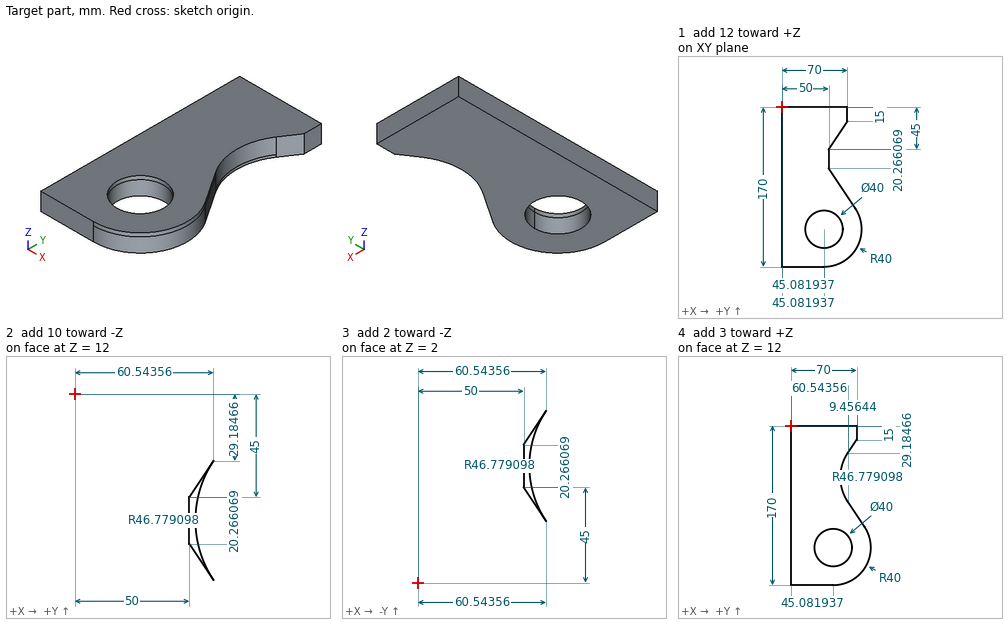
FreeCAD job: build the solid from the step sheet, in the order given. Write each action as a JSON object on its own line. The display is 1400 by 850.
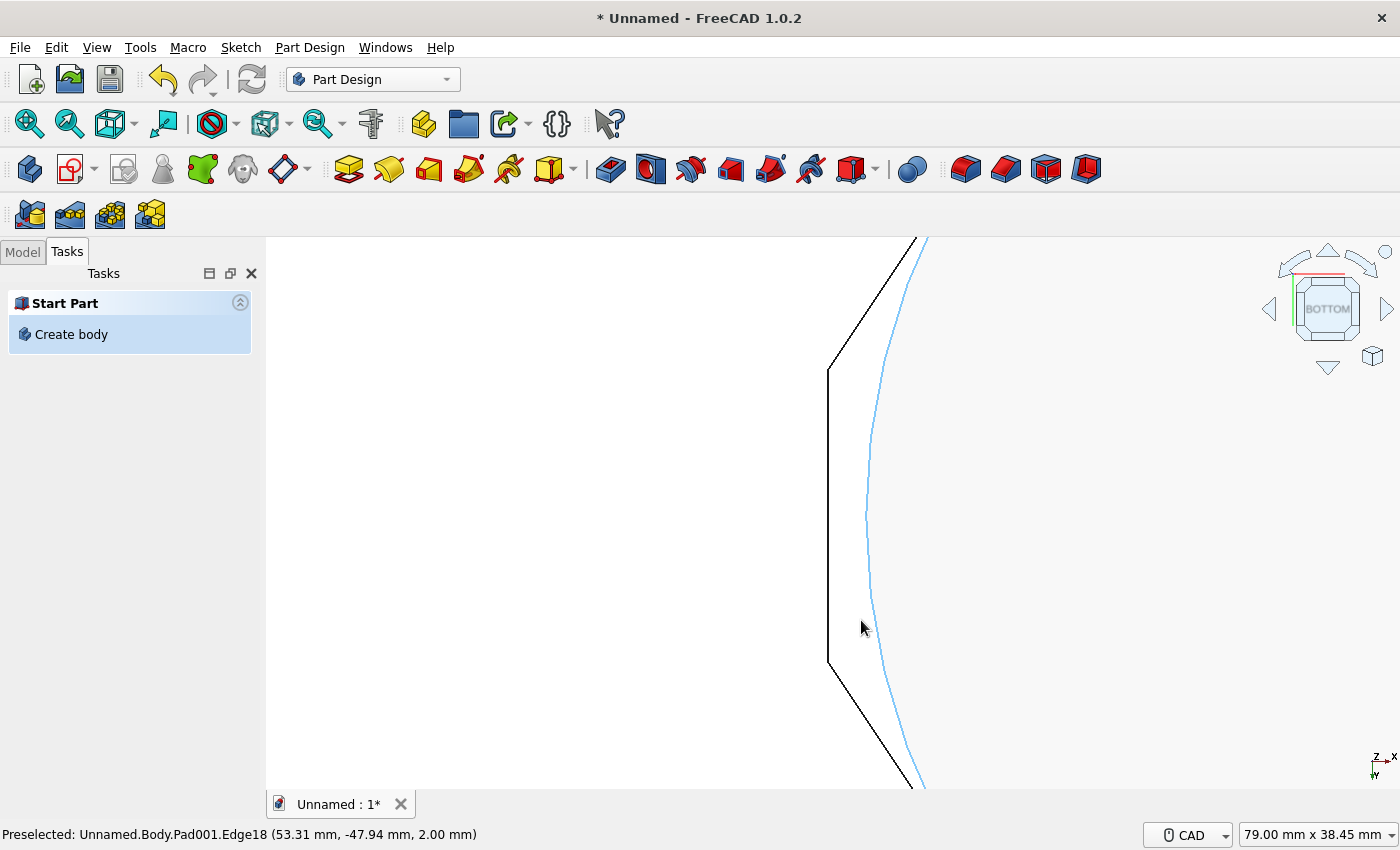
{"action": "left_click", "coordinate": [860, 621]}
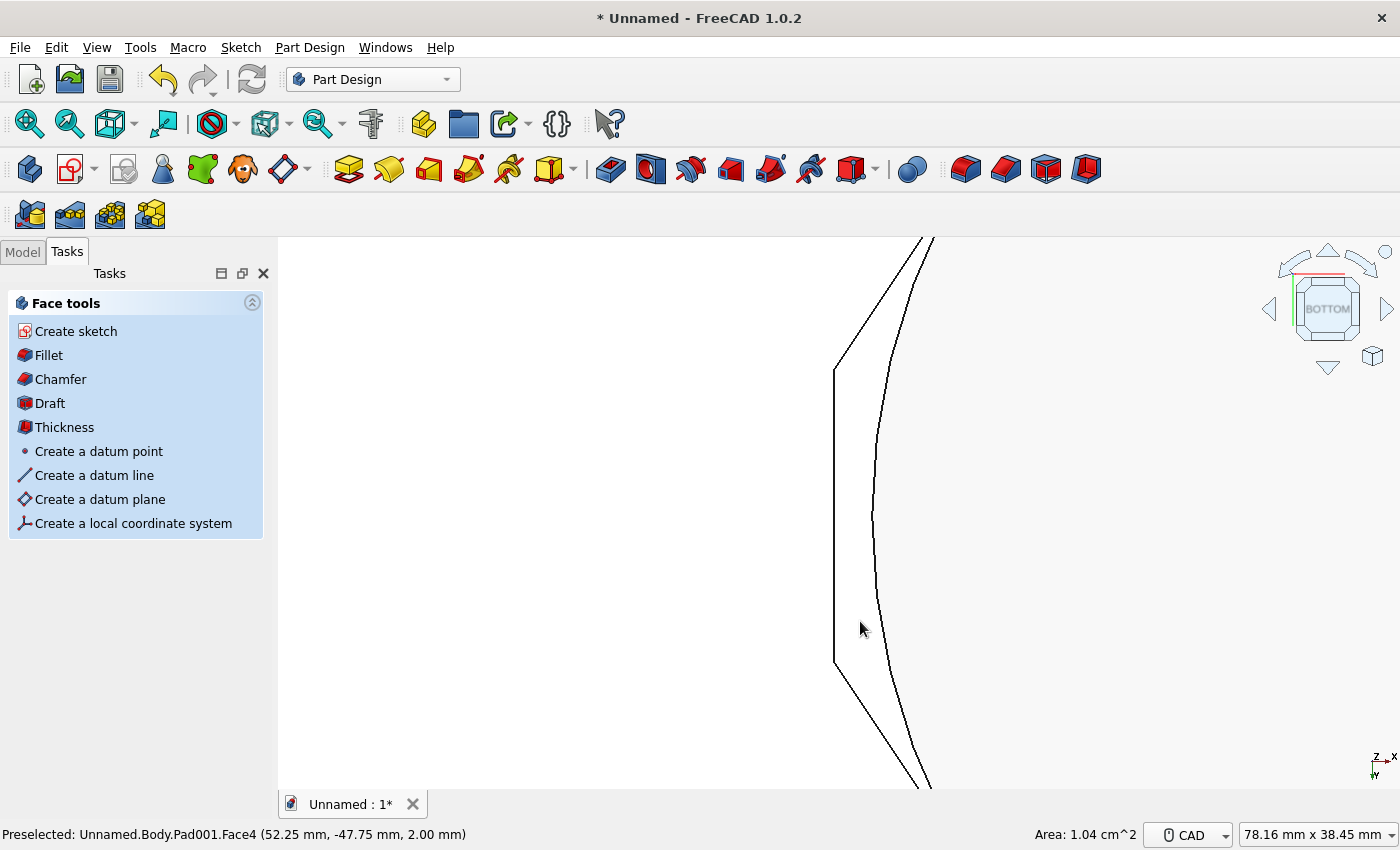
{"action": "left_click", "coordinate": [70, 170]}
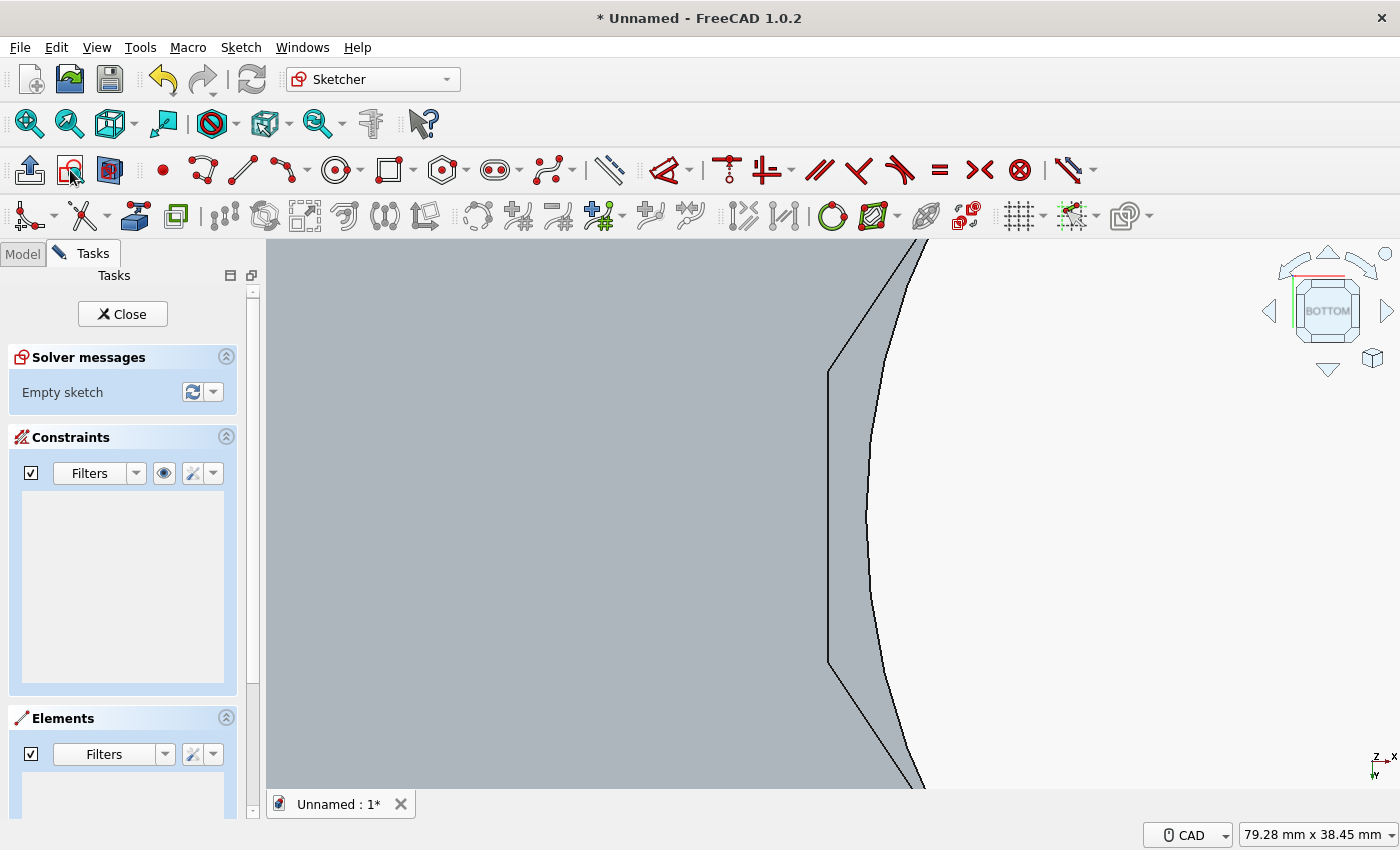
{"action": "scroll", "coordinate": [859, 423], "scroll_direction": "down", "scroll_amount": 6}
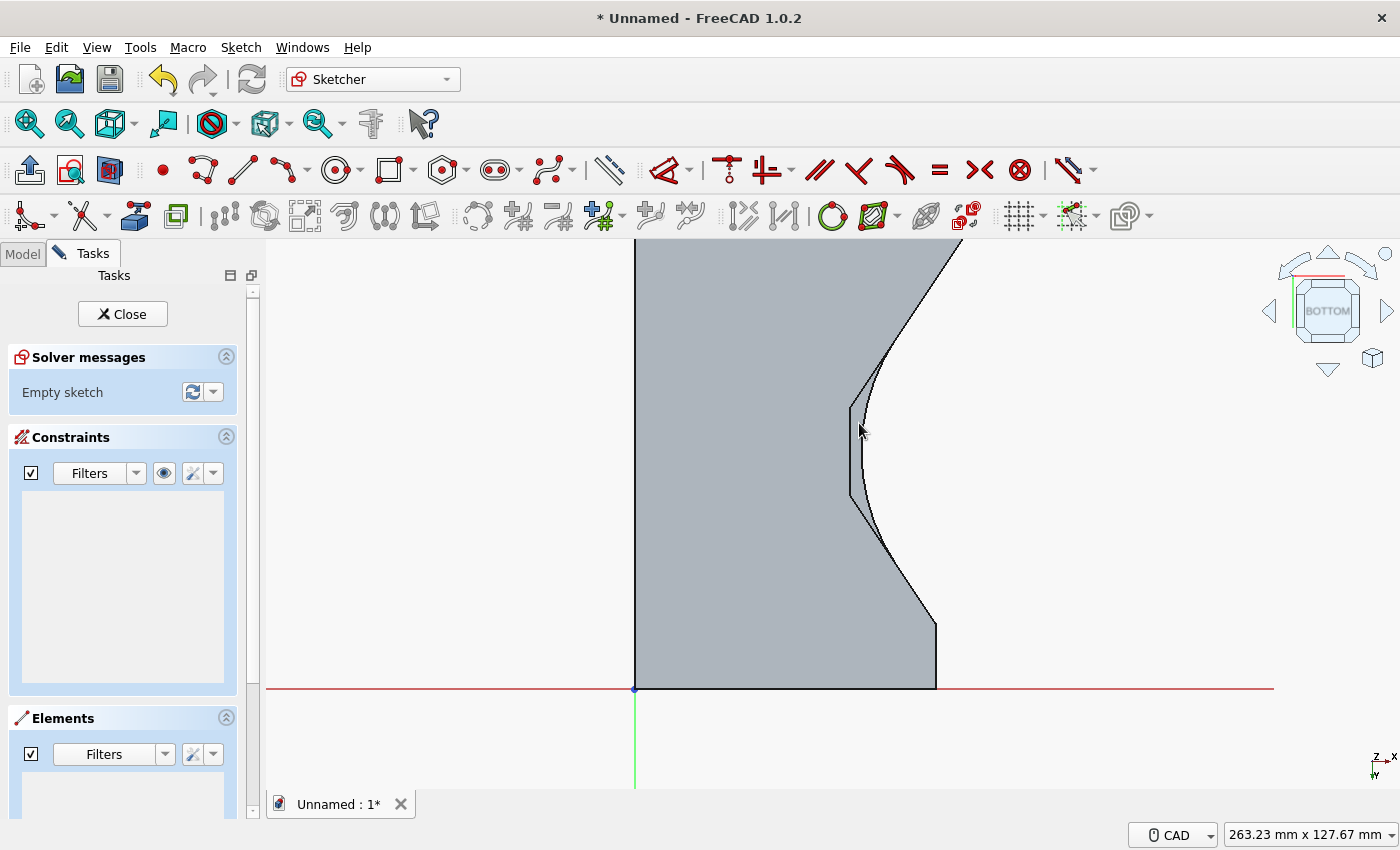
{"action": "left_click", "coordinate": [204, 170]}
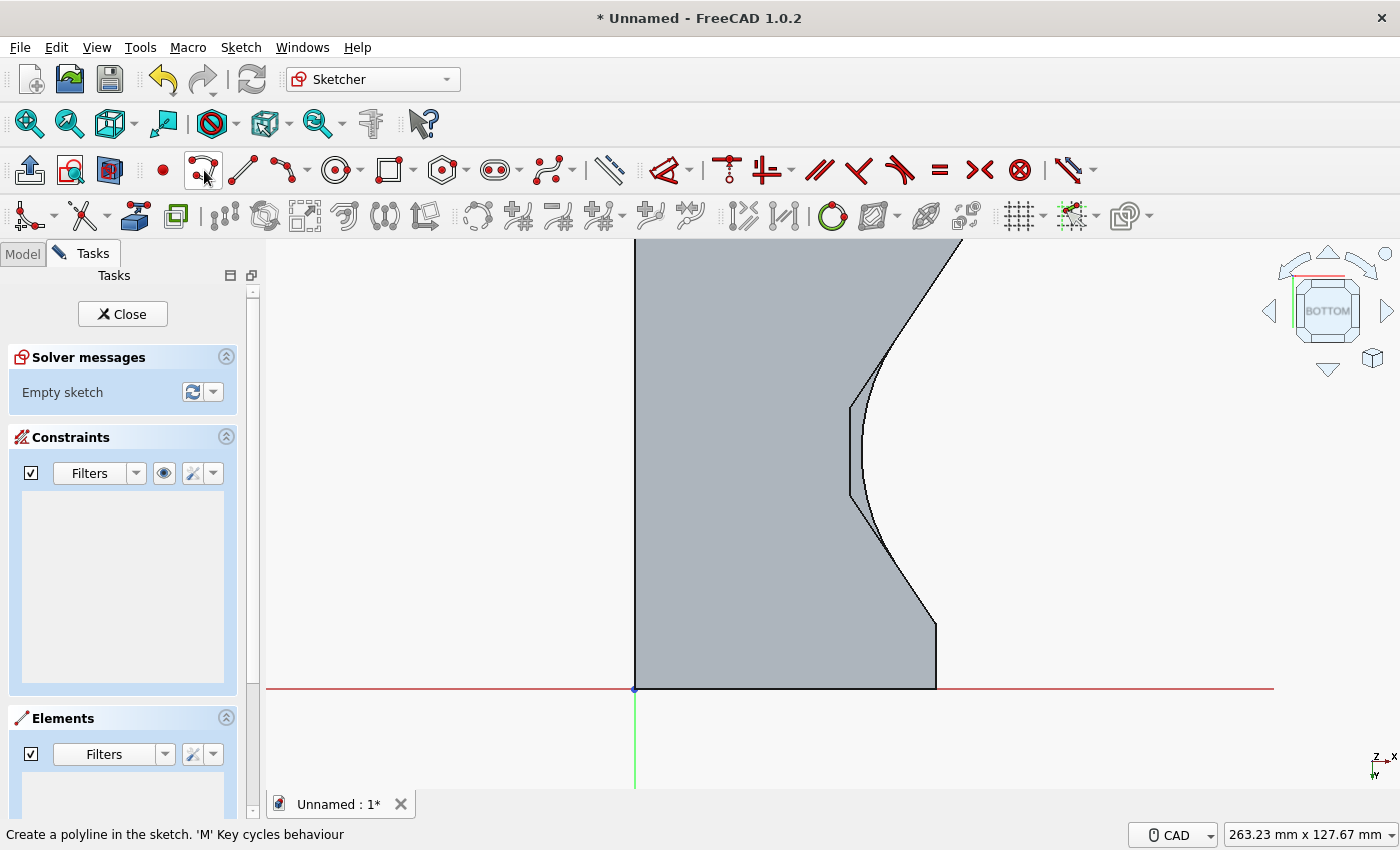
{"action": "left_click", "coordinate": [895, 340]}
{"action": "left_click", "coordinate": [850, 408]}
{"action": "left_click", "coordinate": [850, 495]}
{"action": "left_click", "coordinate": [895, 563]}
{"action": "right_click", "coordinate": [895, 563]}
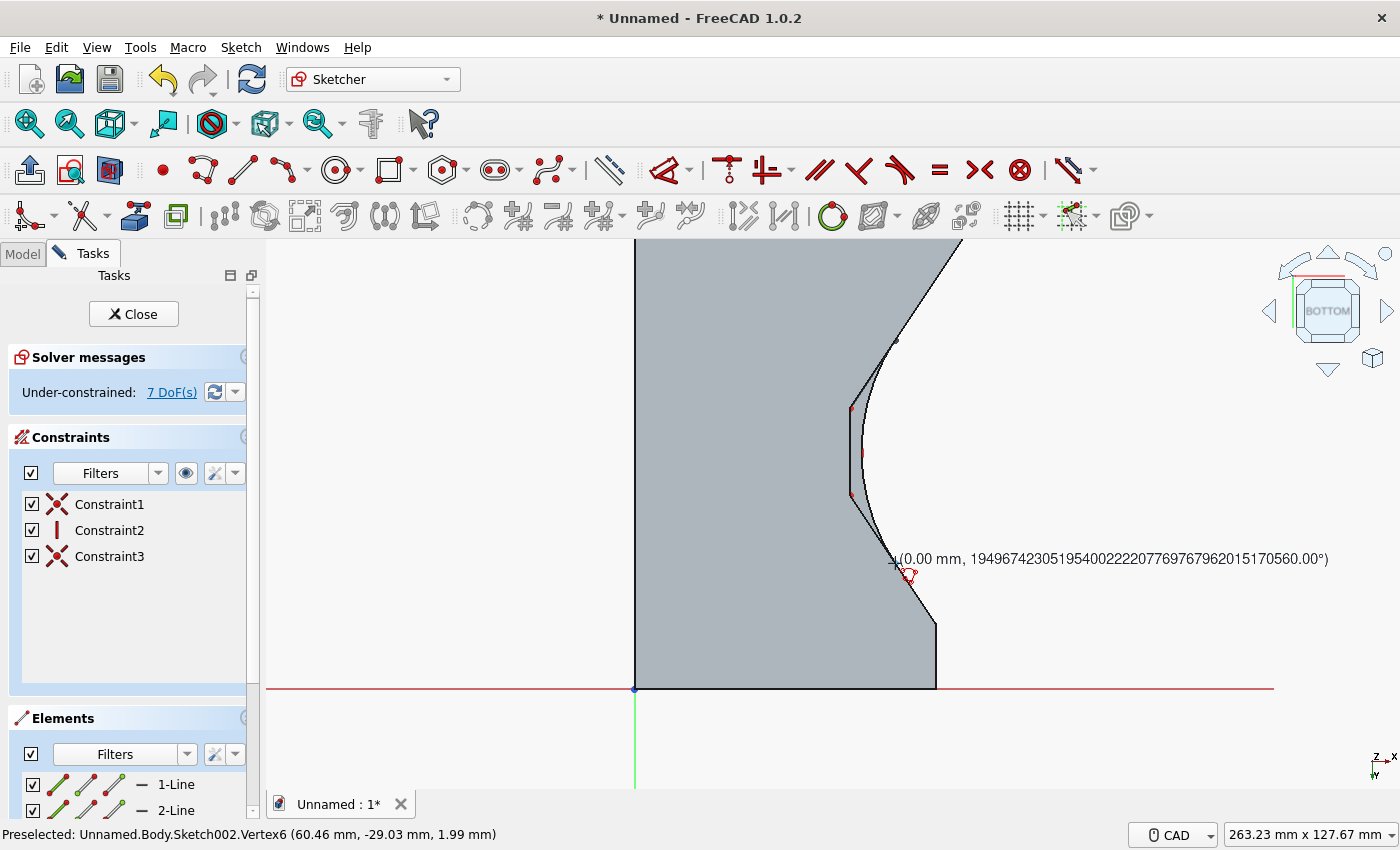
{"action": "left_click", "coordinate": [284, 170]}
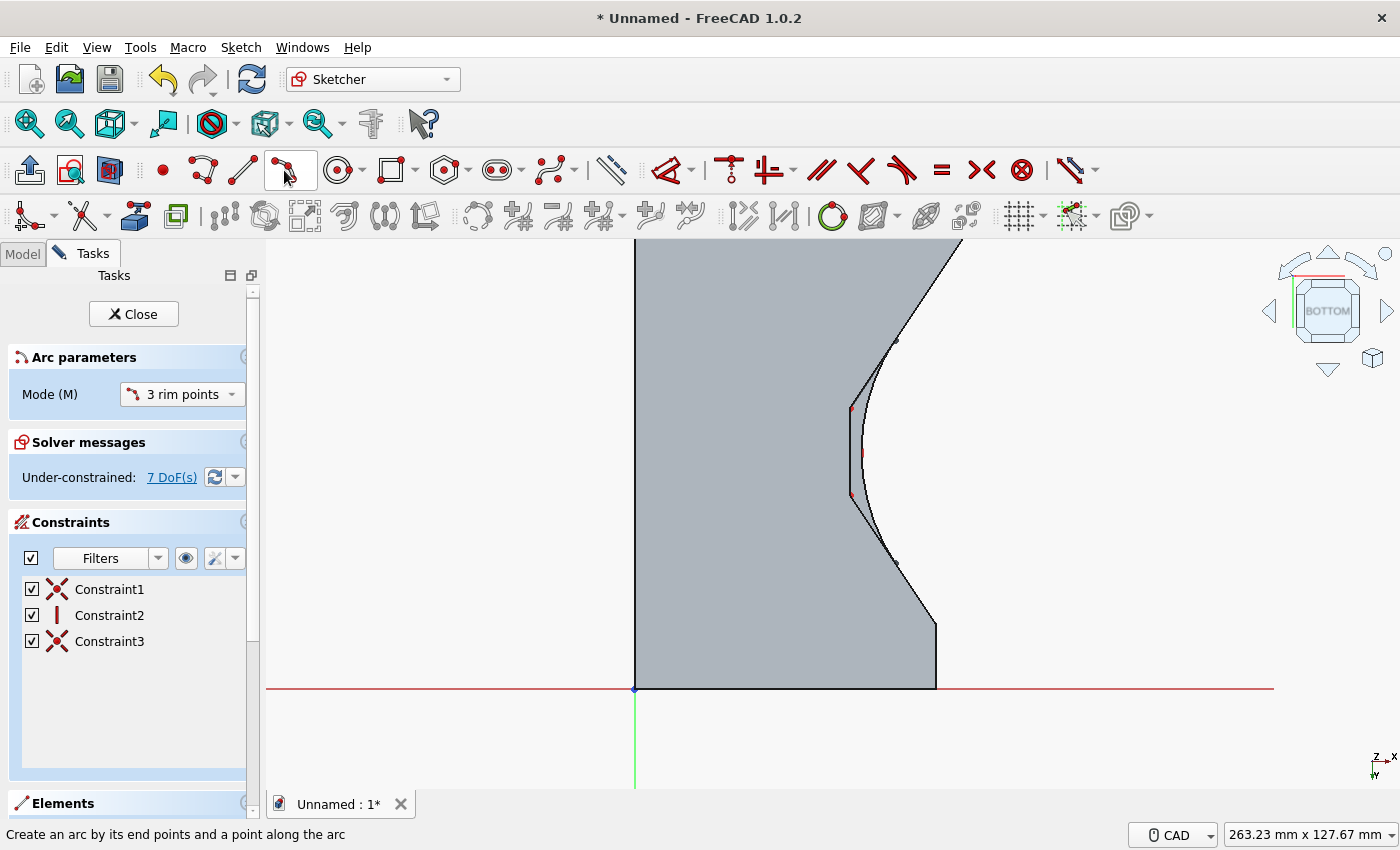
{"action": "left_click", "coordinate": [895, 564]}
{"action": "left_click", "coordinate": [895, 341]}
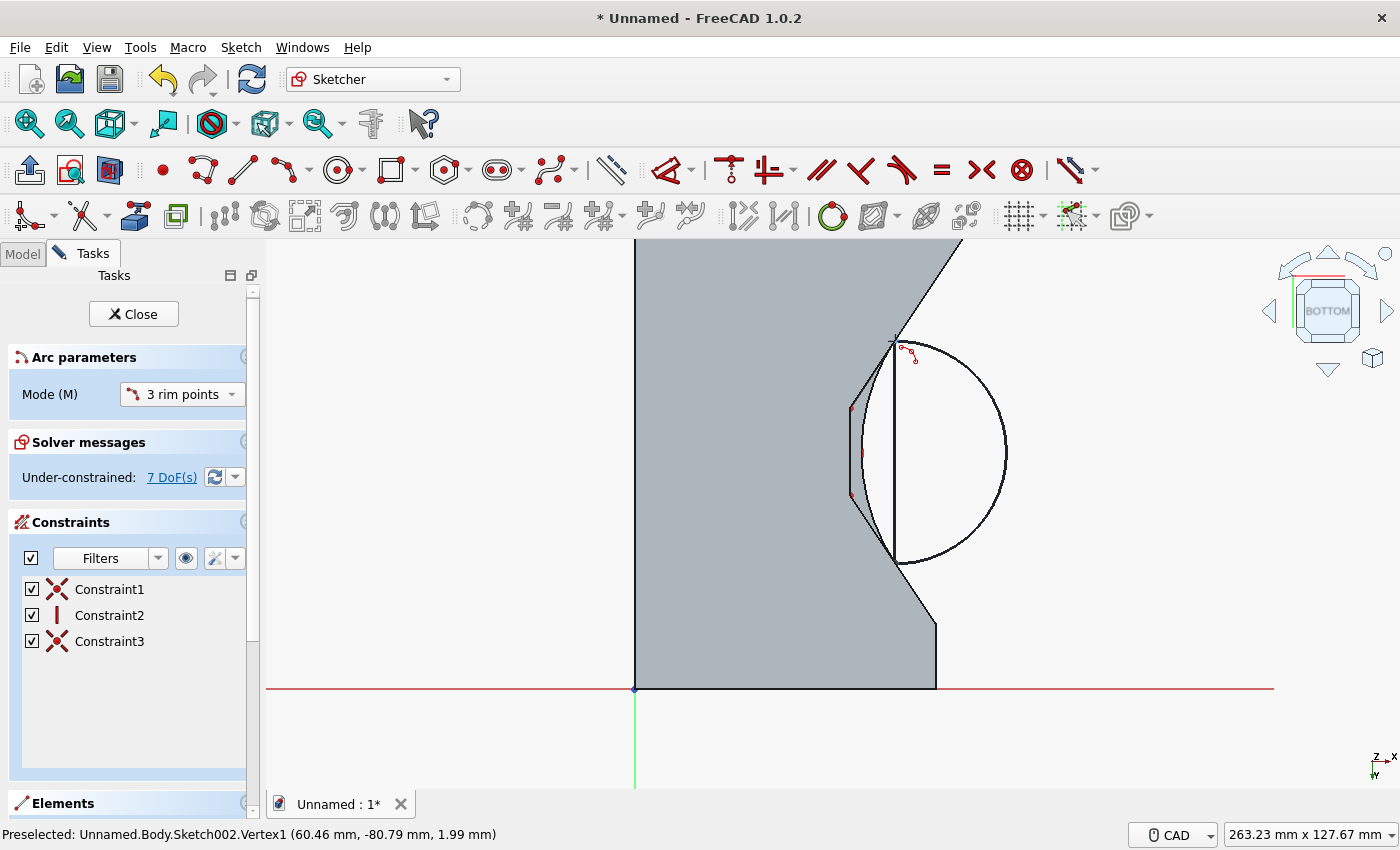
{"action": "scroll", "coordinate": [863, 428], "scroll_direction": "up", "scroll_amount": 2}